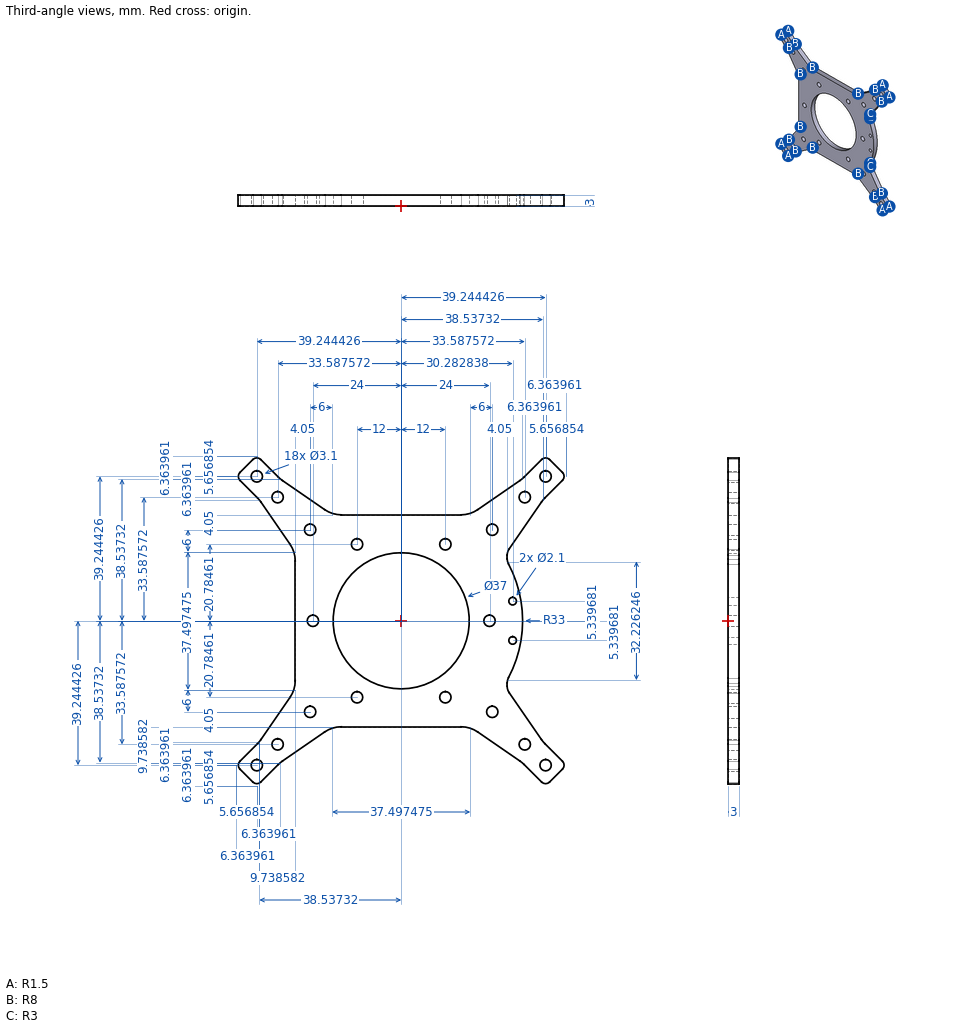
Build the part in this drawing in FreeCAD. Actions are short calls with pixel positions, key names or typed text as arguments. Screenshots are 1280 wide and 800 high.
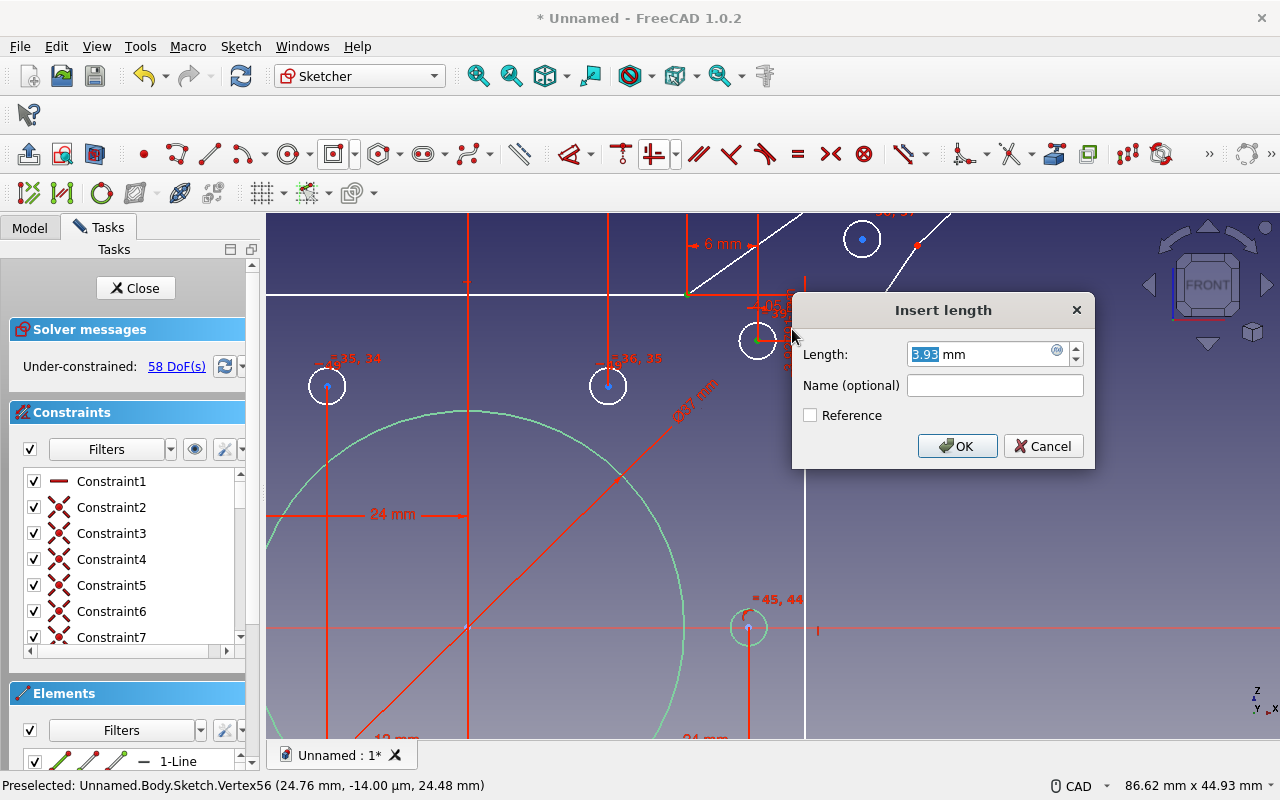
text(4.05)
key(Return)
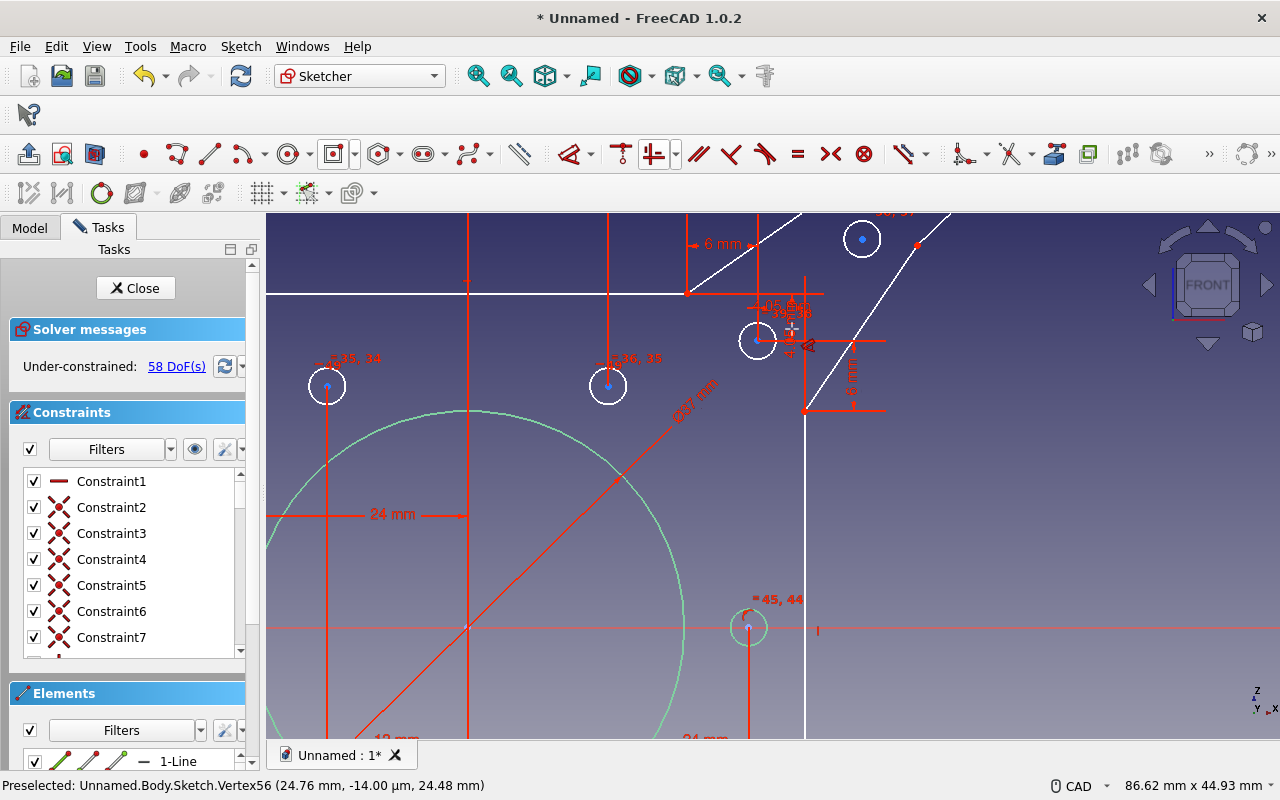
scroll(807, 411, down, 6)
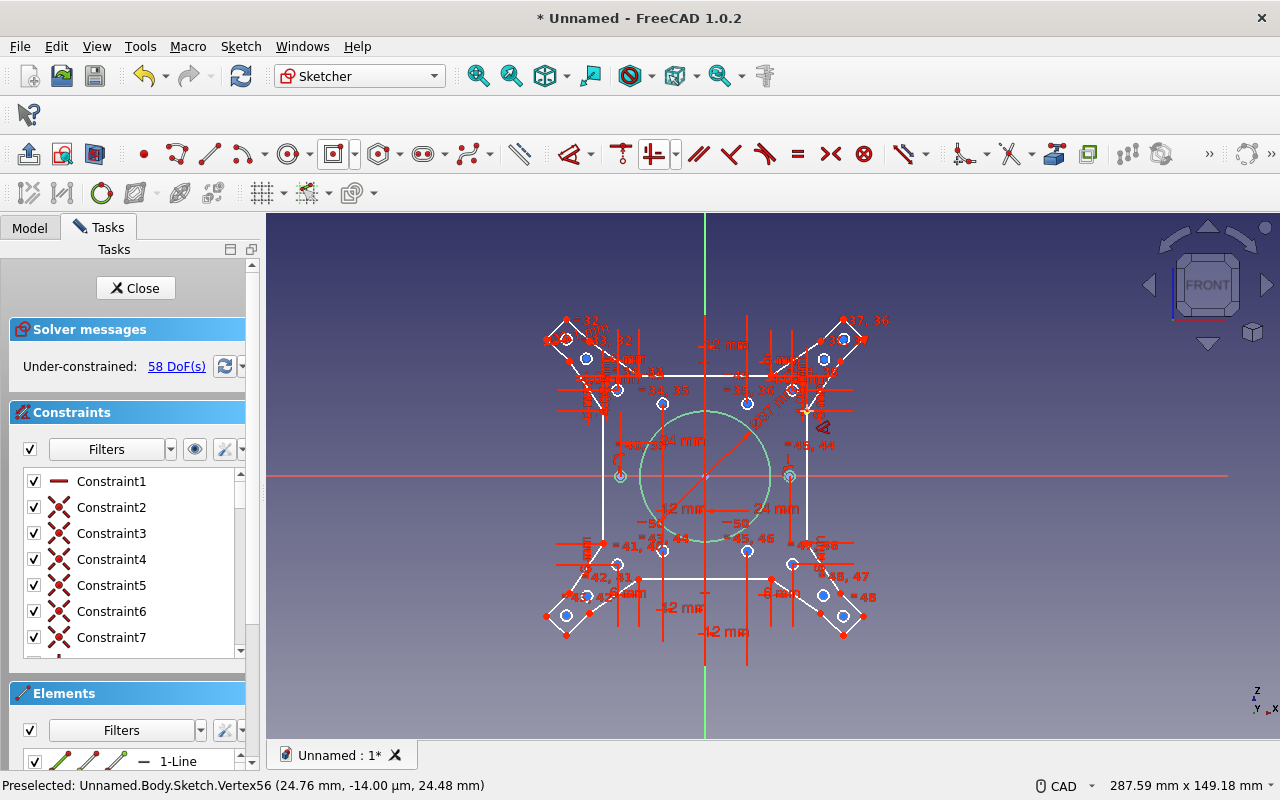
scroll(603, 544, up, 6)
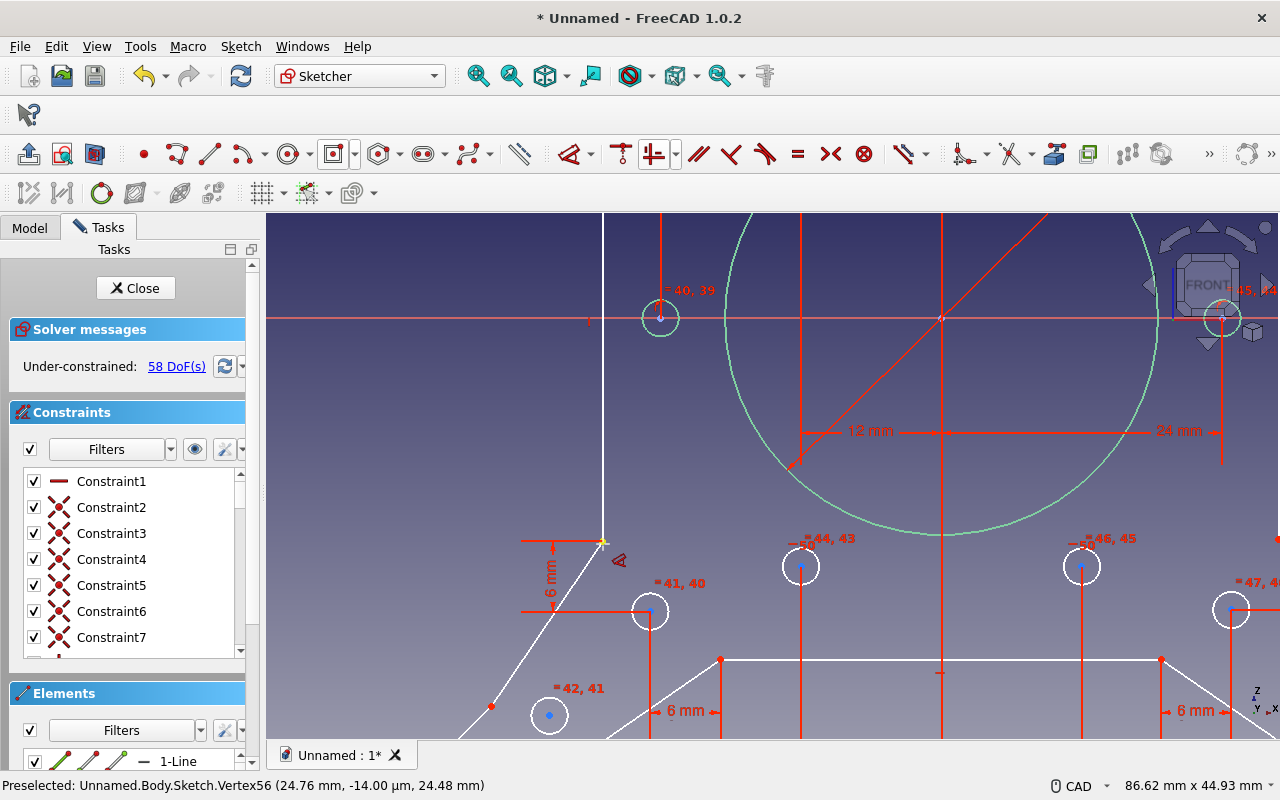
click(603, 541)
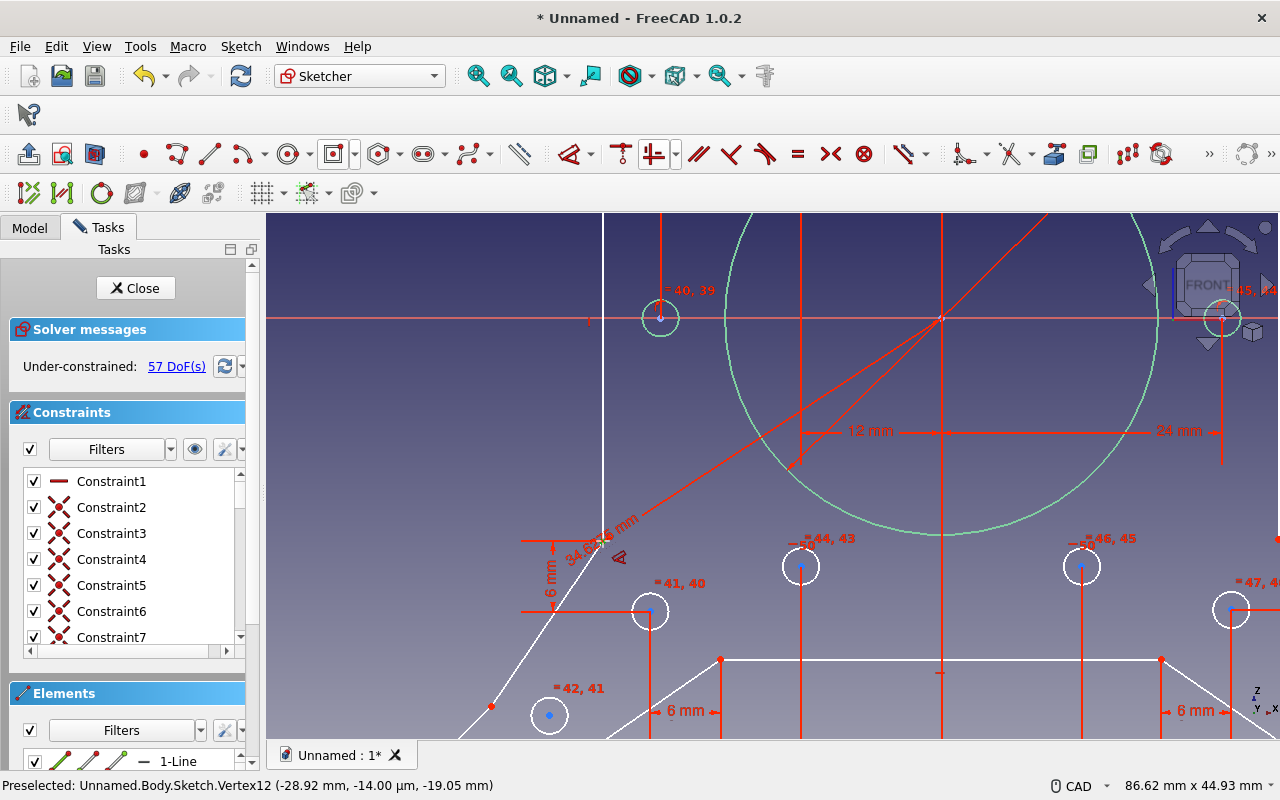
click(650, 612)
click(627, 646)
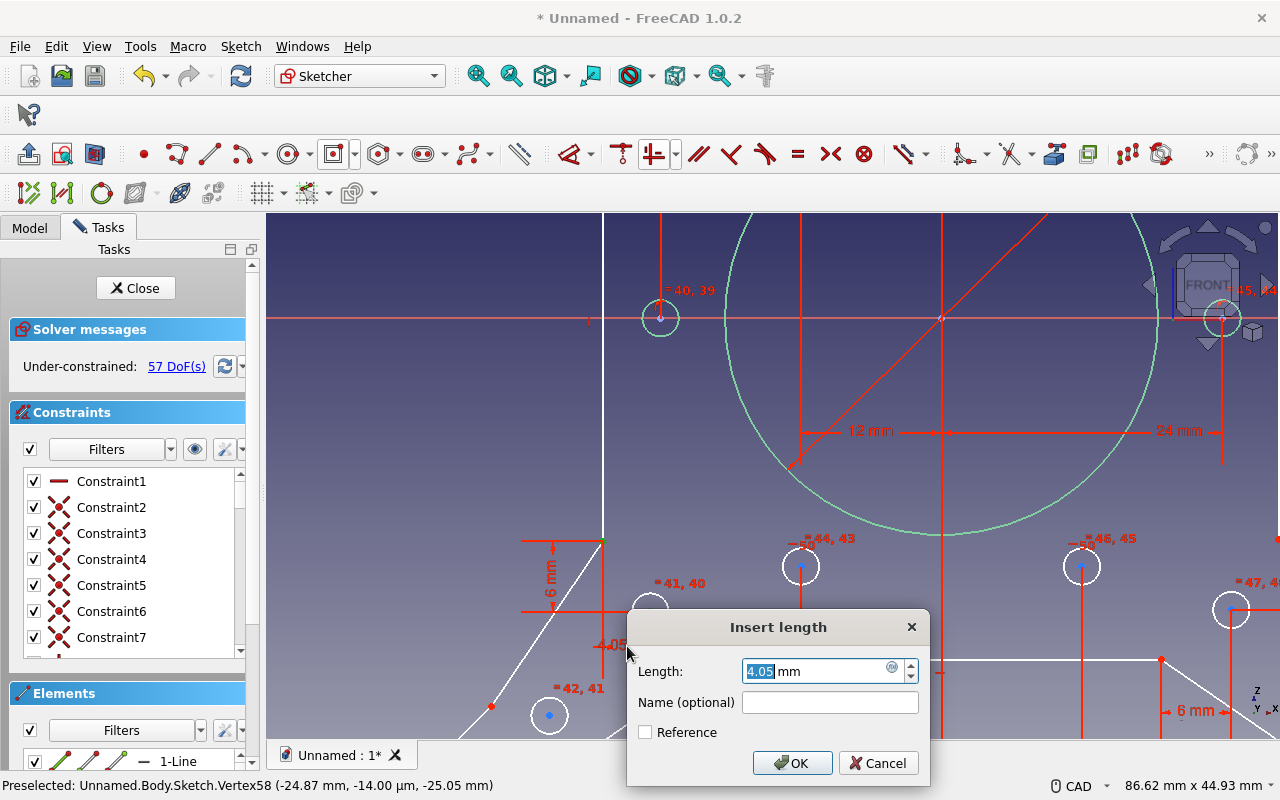
text(4.05)
key(Return)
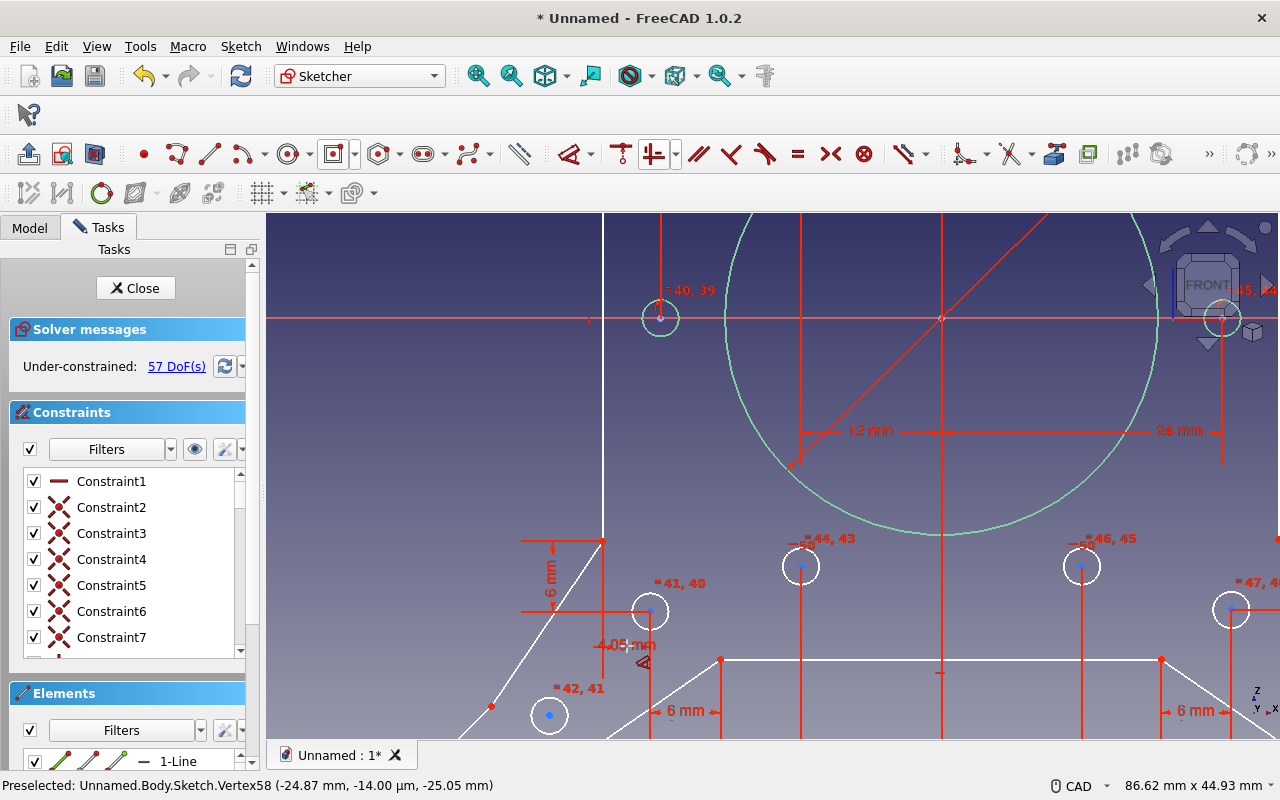
click(721, 660)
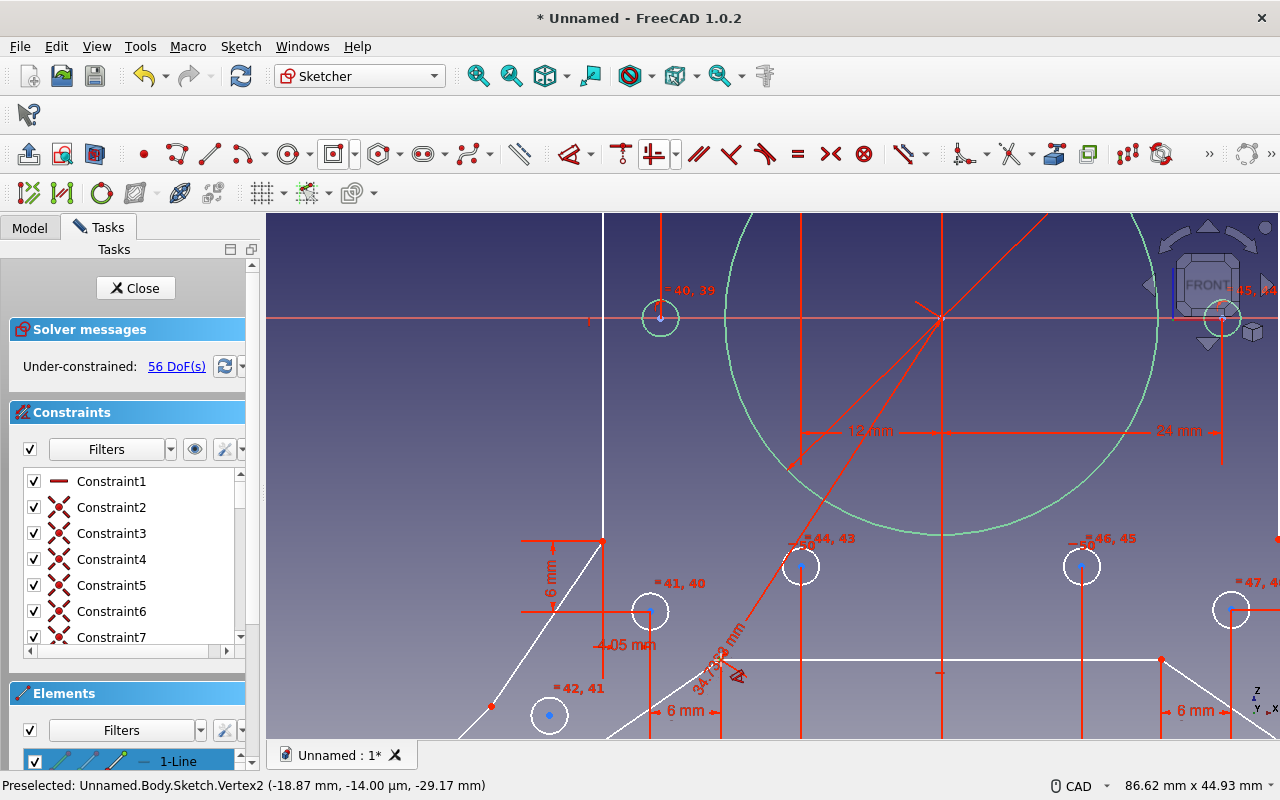
click(650, 612)
click(616, 625)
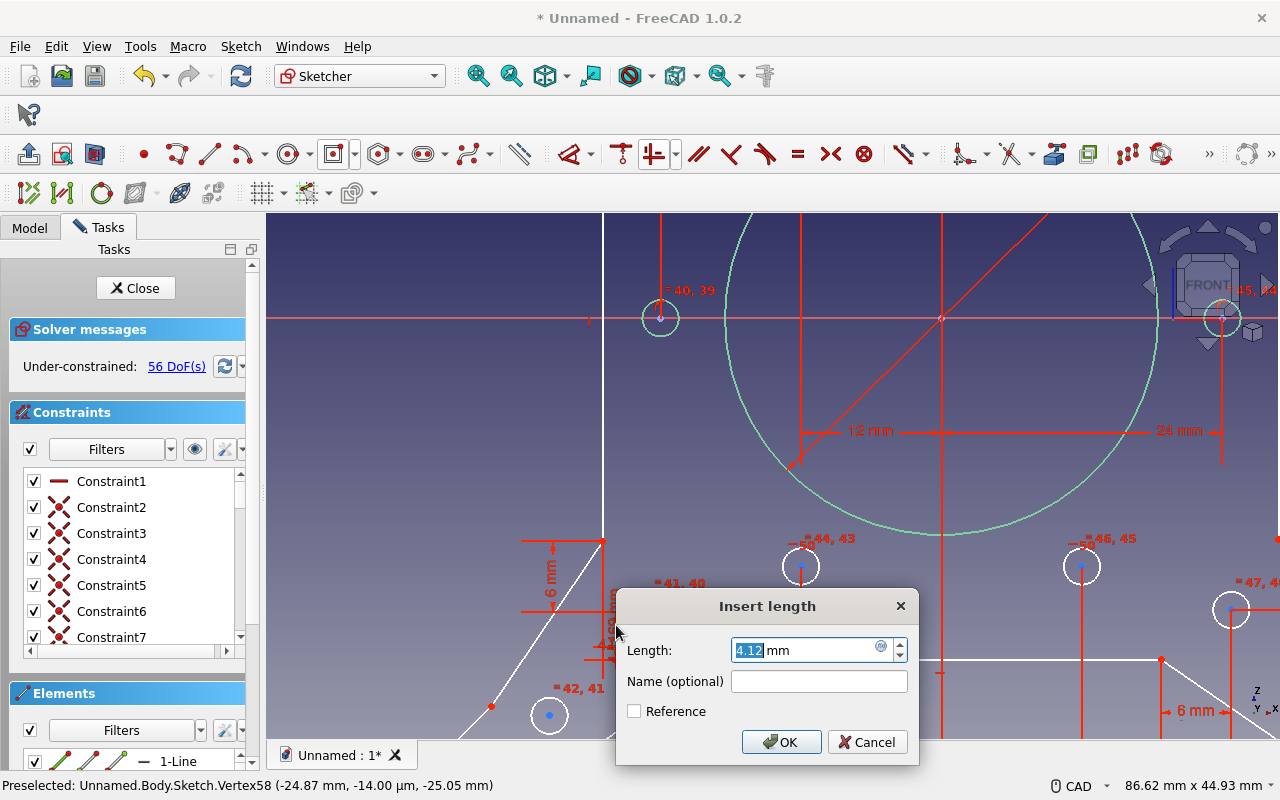
text(4.05)
key(Return)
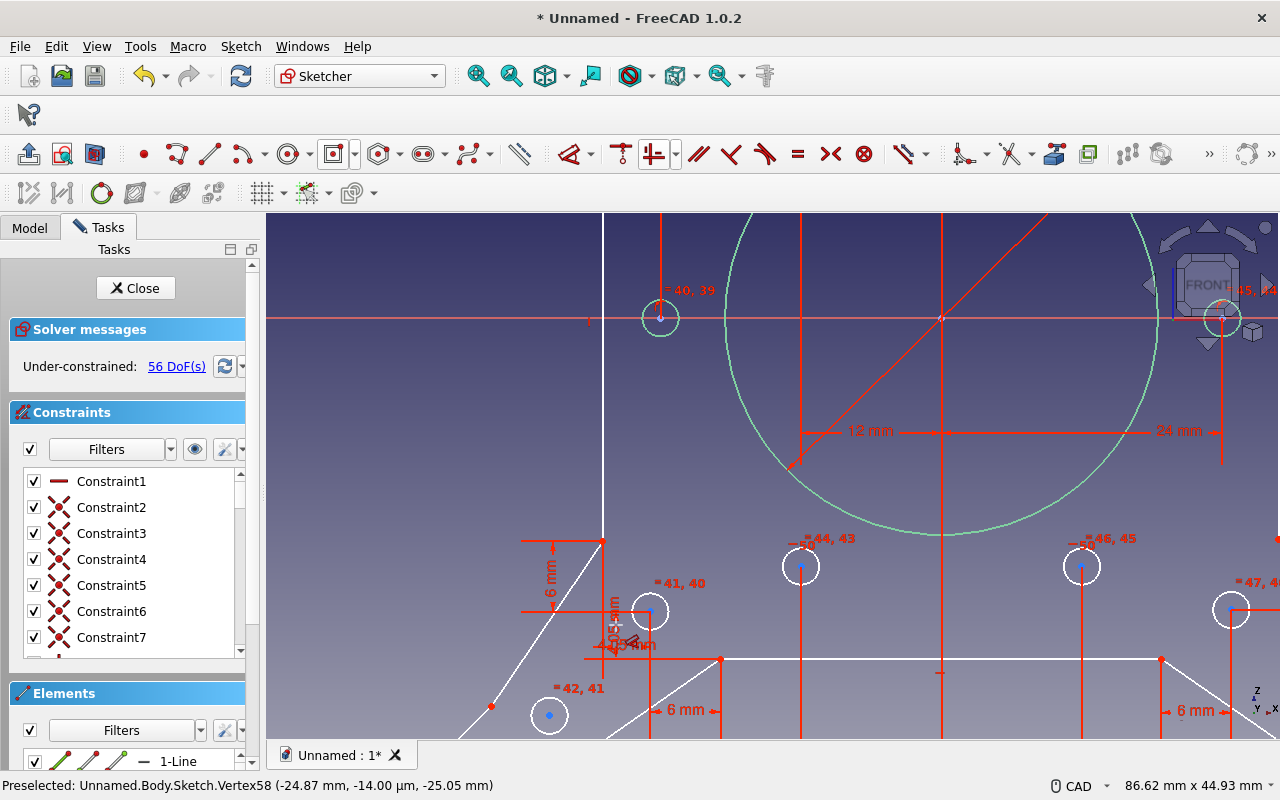
scroll(602, 544, down, 6)